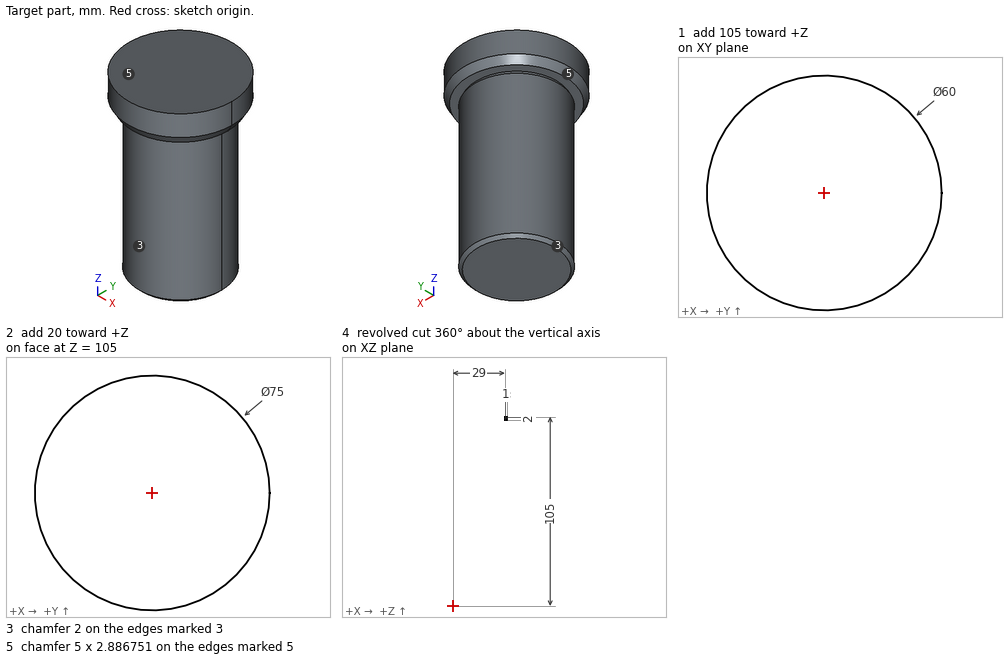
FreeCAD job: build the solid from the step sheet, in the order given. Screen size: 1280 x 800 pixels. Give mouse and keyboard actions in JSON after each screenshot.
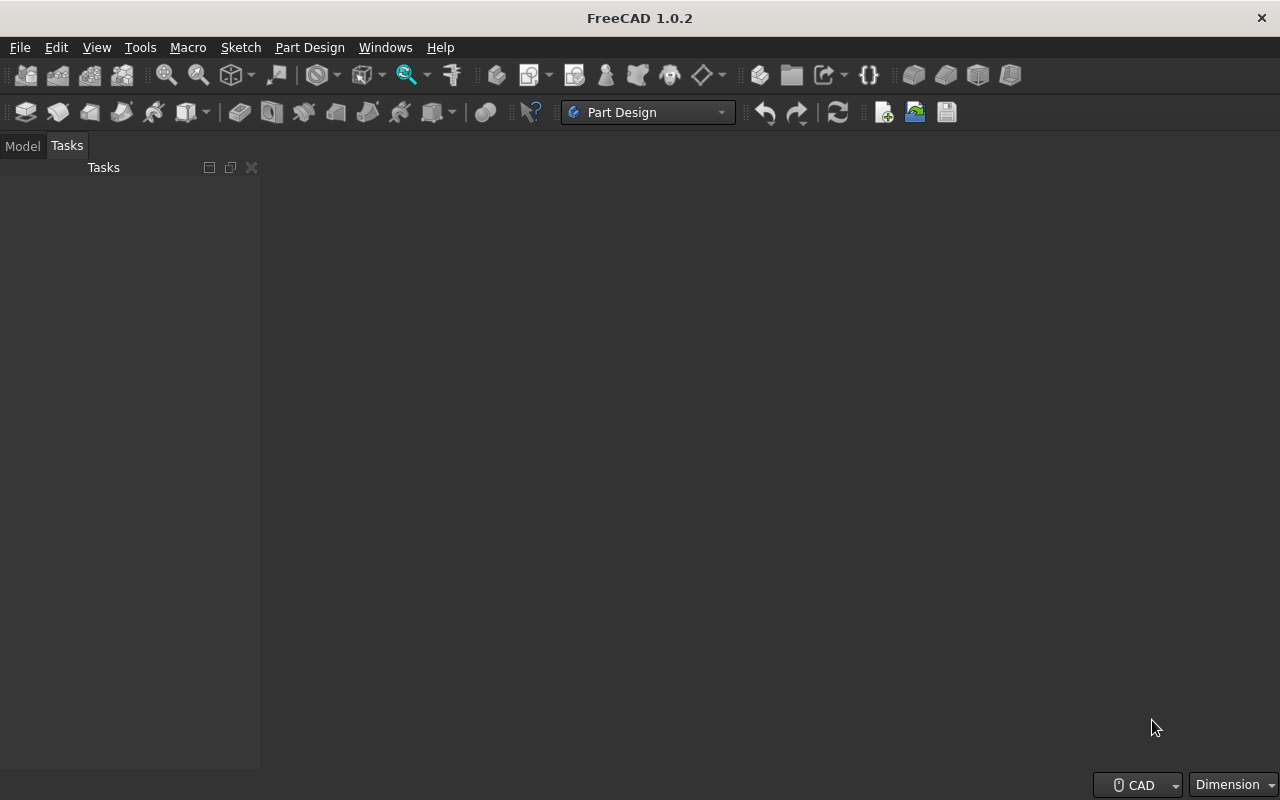
{"action": "left_click", "coordinate": [884, 112]}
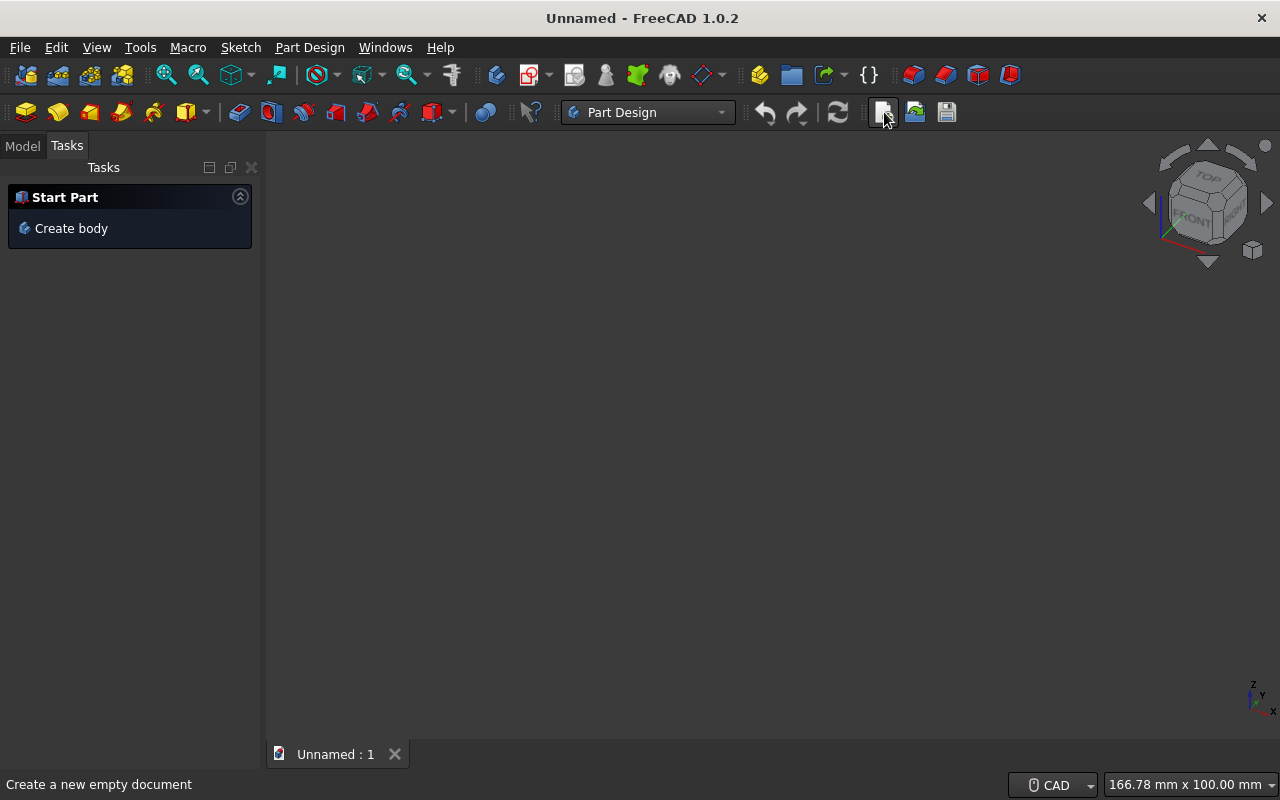
{"action": "left_click", "coordinate": [530, 76]}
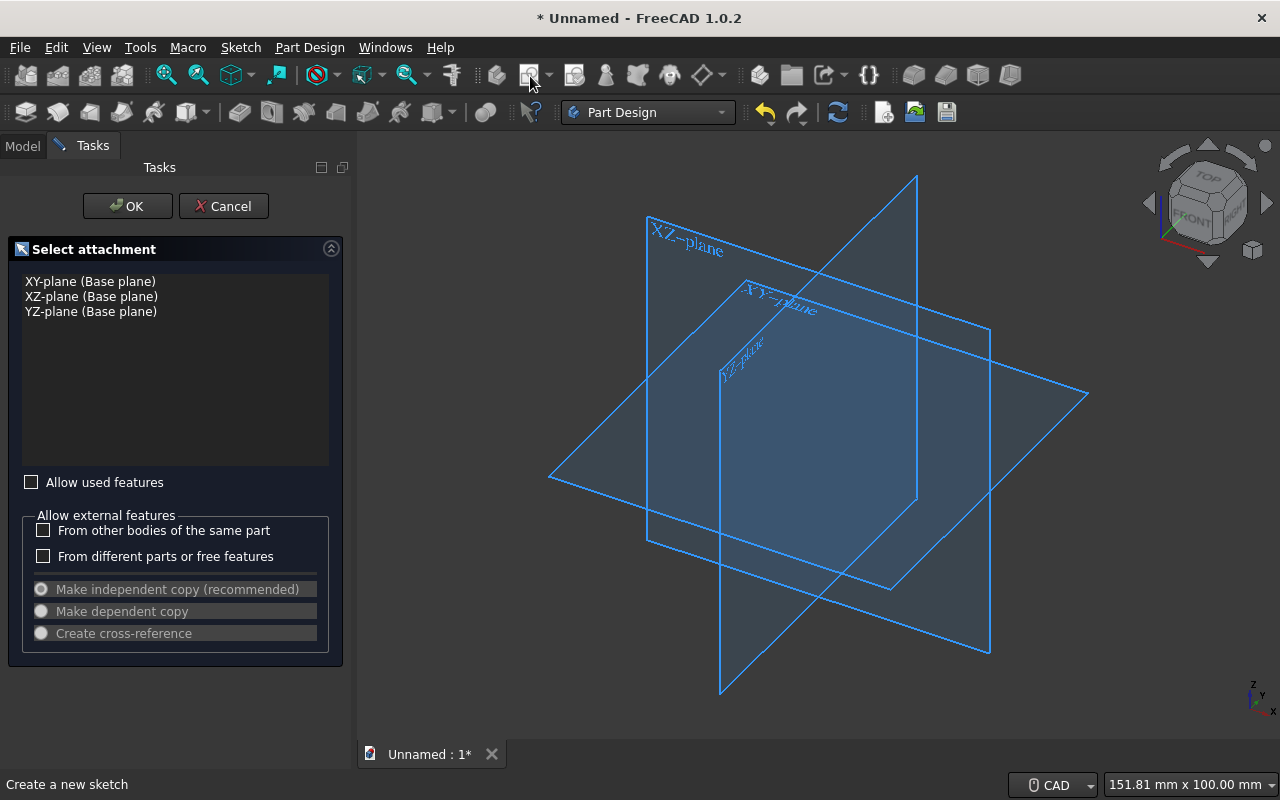
{"action": "left_click", "coordinate": [82, 282]}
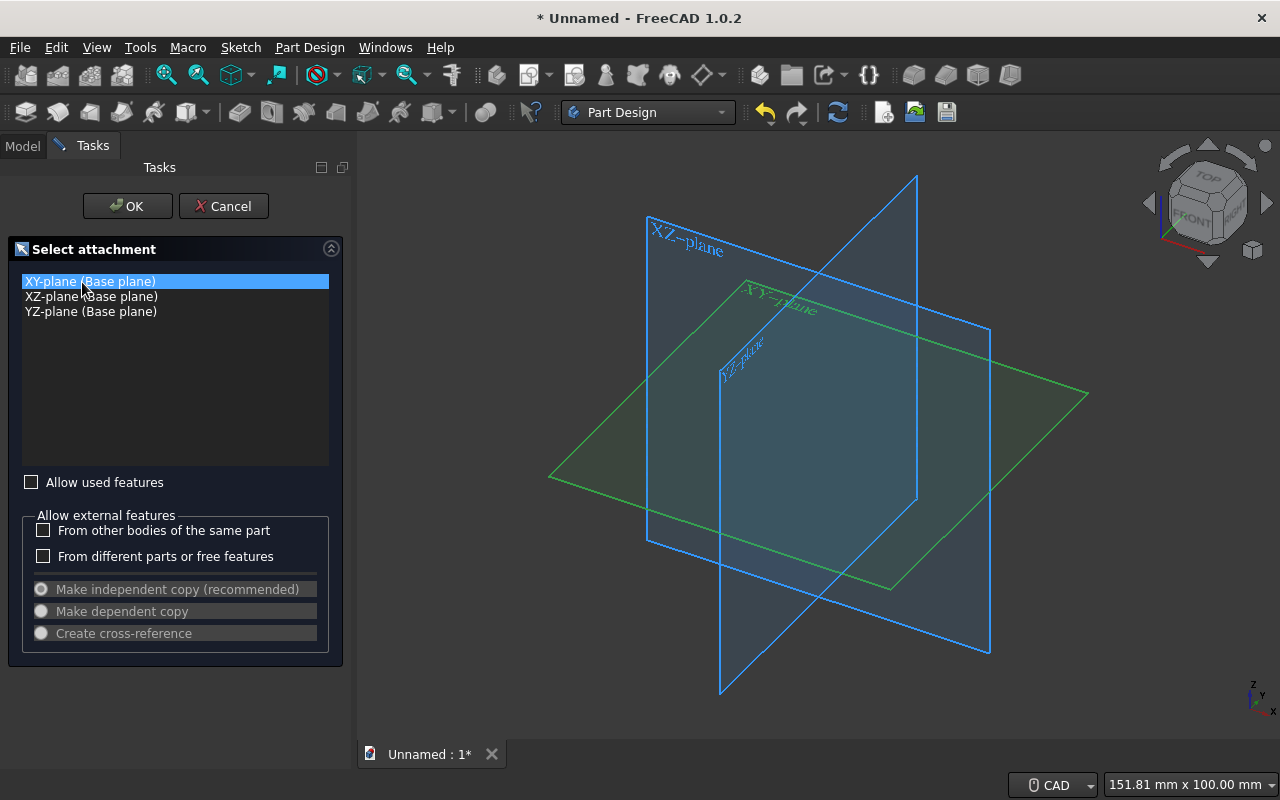
{"action": "left_click", "coordinate": [128, 206]}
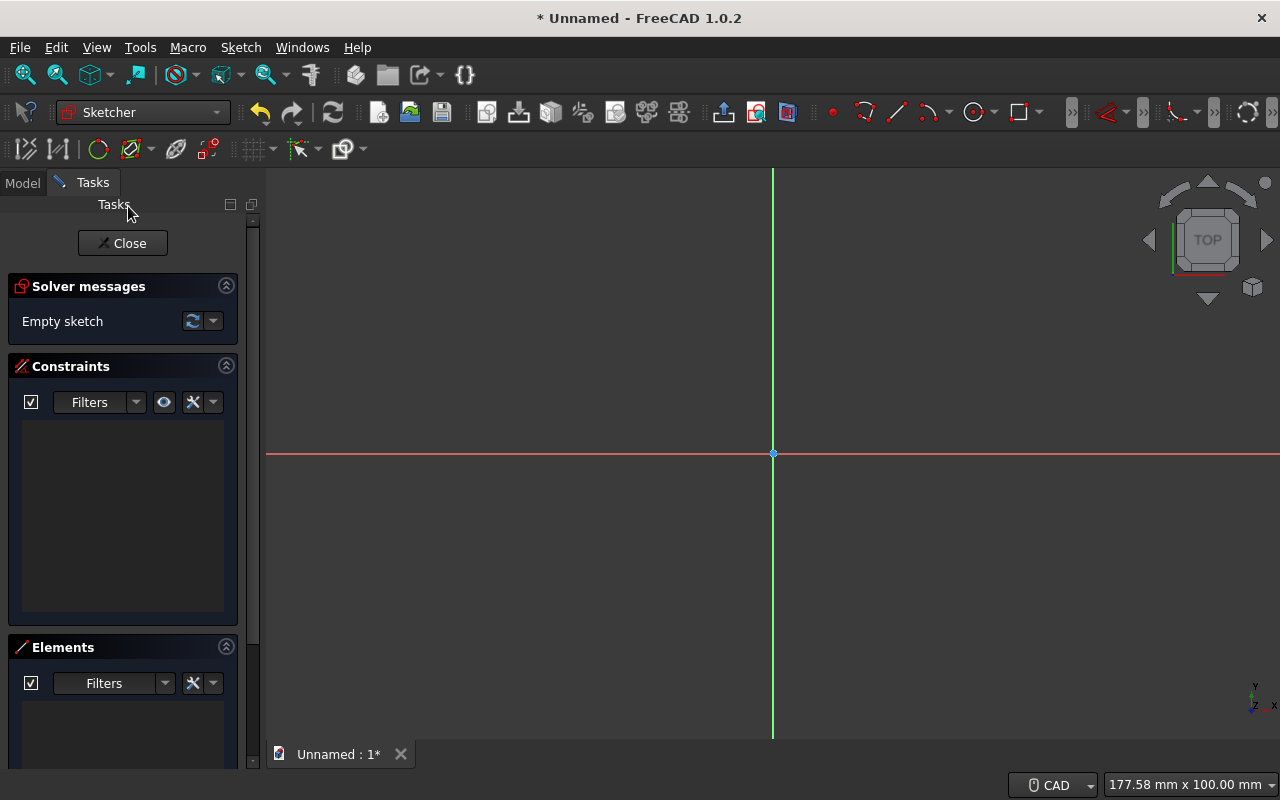
{"action": "left_click", "coordinate": [974, 112]}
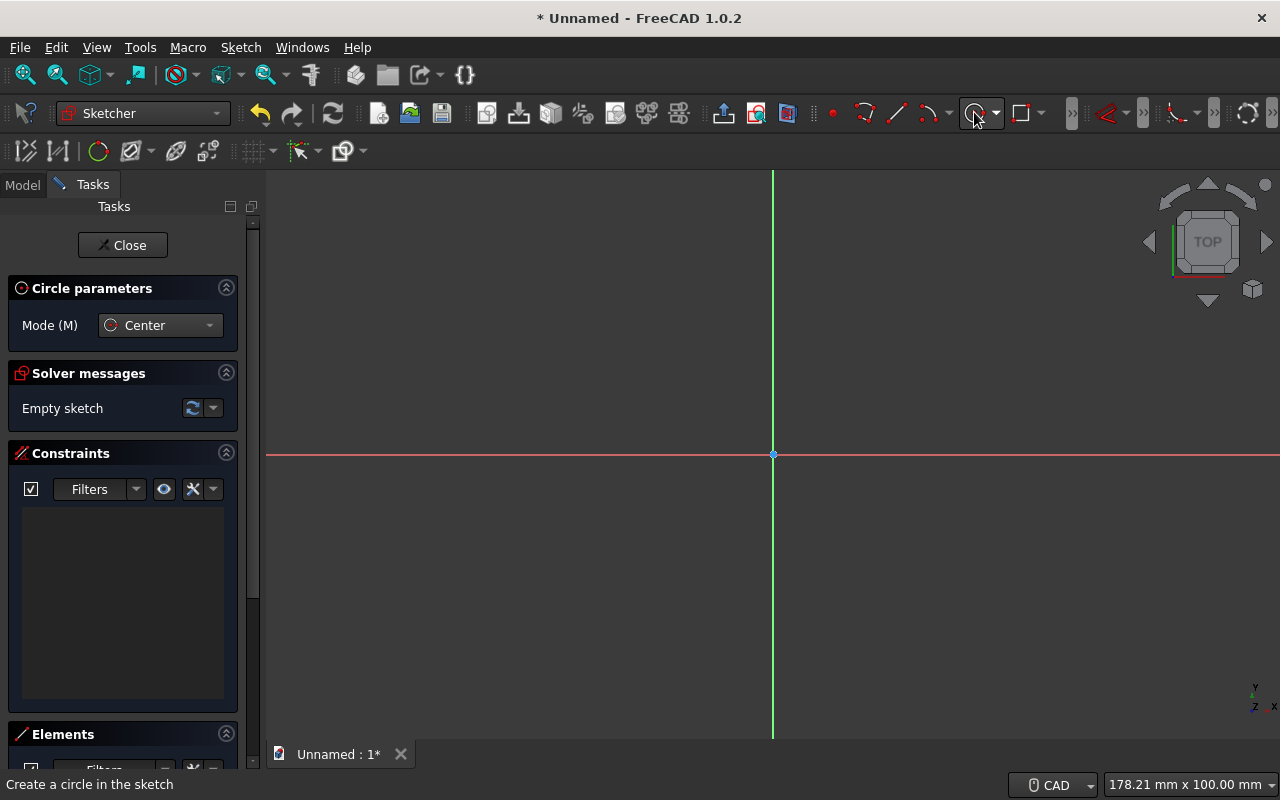
{"action": "left_click", "coordinate": [773, 454]}
{"action": "mouse_move", "coordinate": [894, 334]}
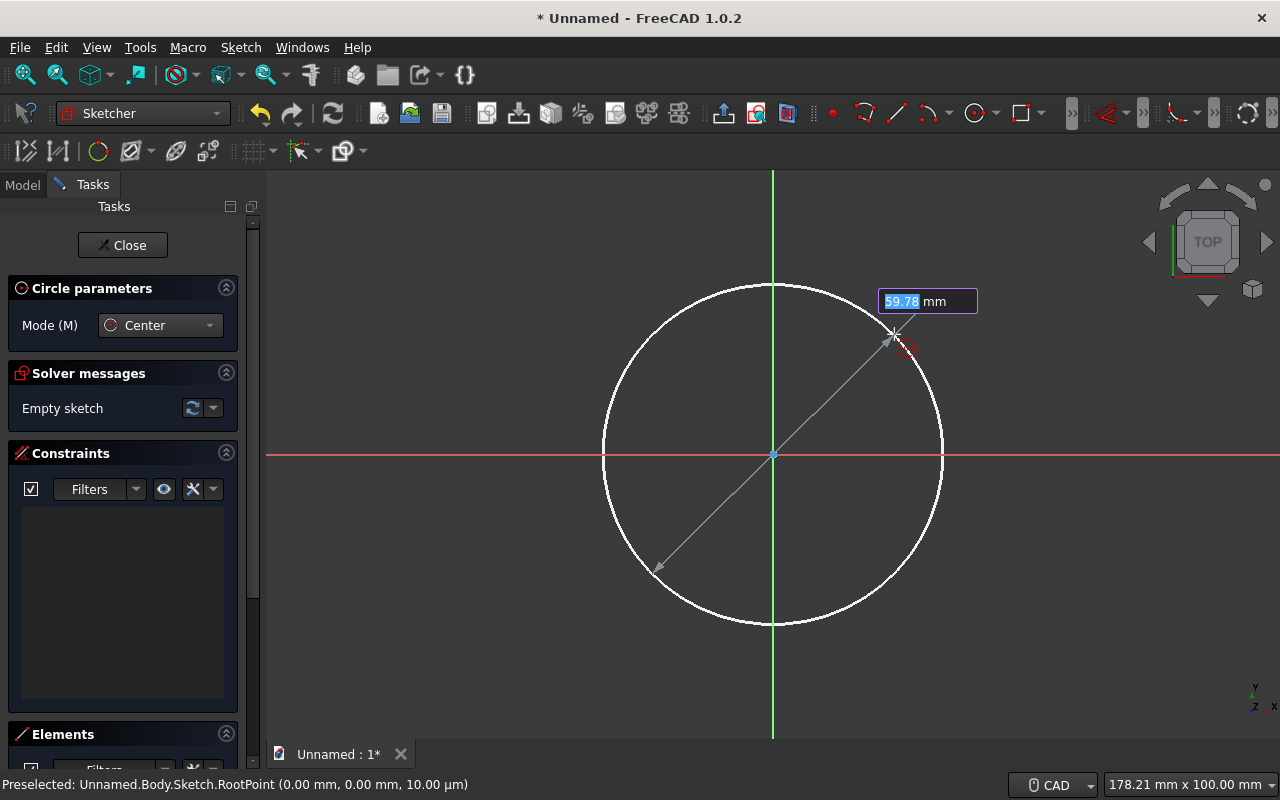
{"action": "type", "text": "60"}
{"action": "key", "text": "Return"}
{"action": "key", "text": "Escape"}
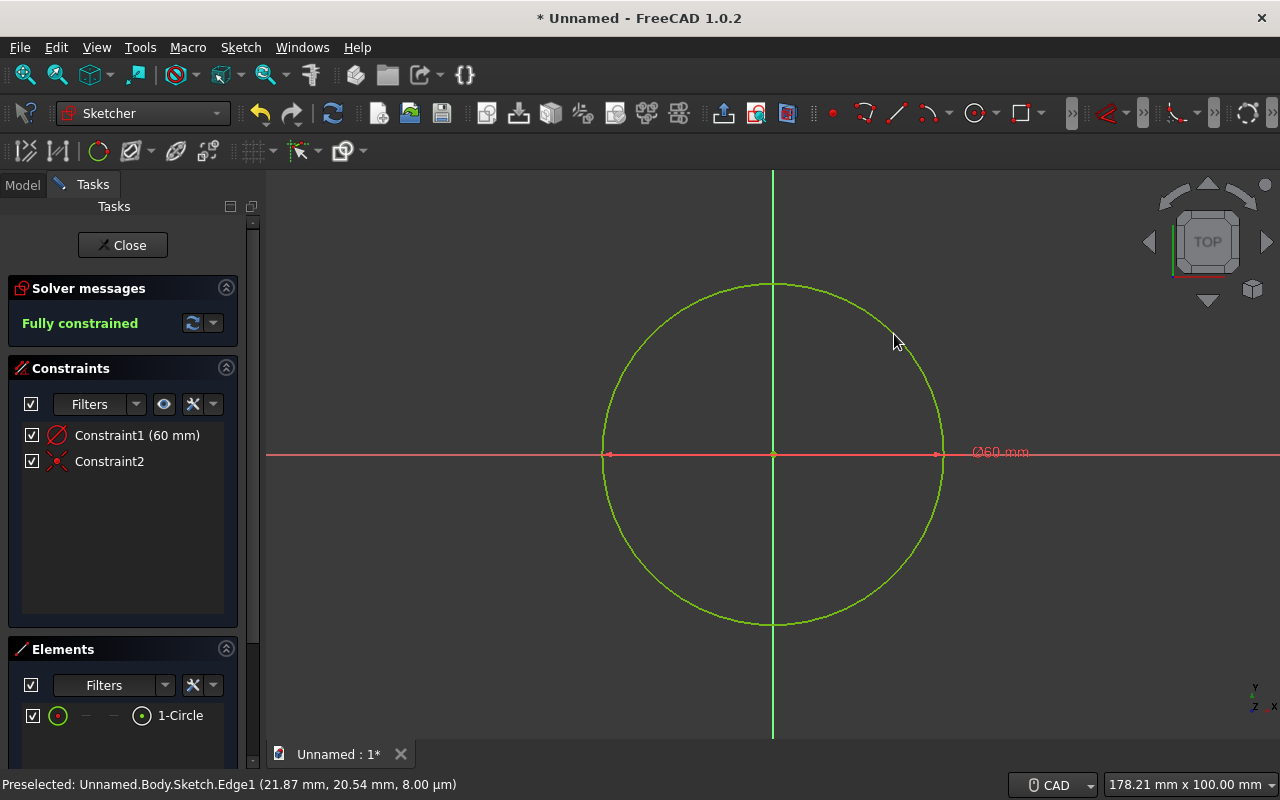
{"action": "left_click", "coordinate": [123, 245]}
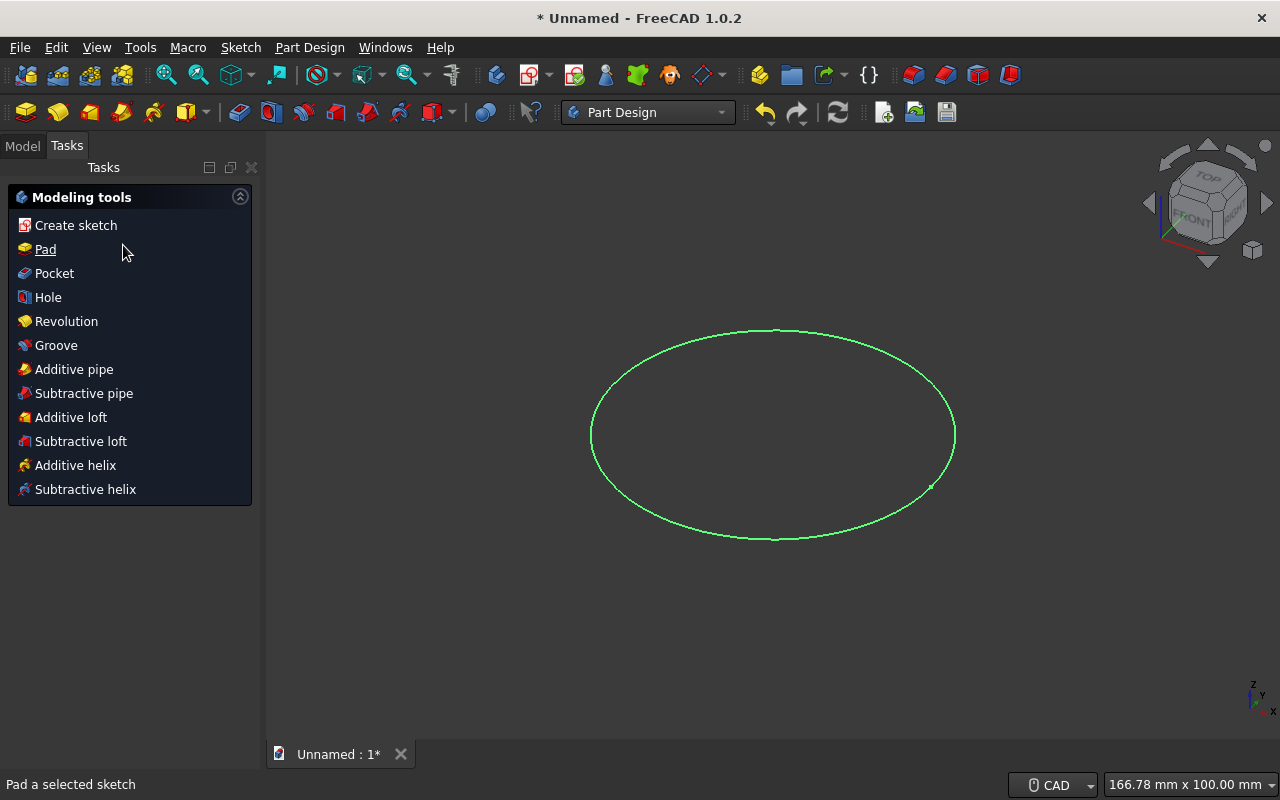
{"action": "left_click", "coordinate": [26, 112]}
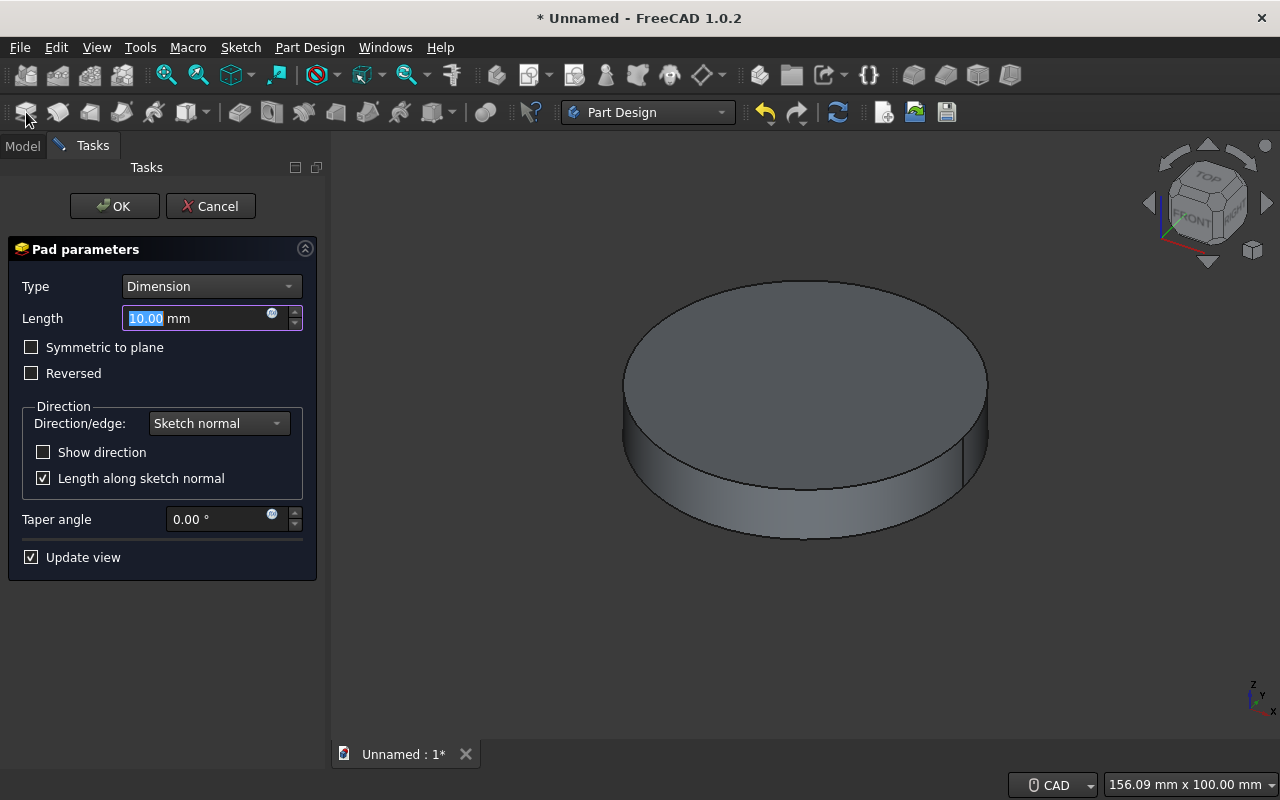
{"action": "type", "text": "105"}
{"action": "key", "text": "Tab"}